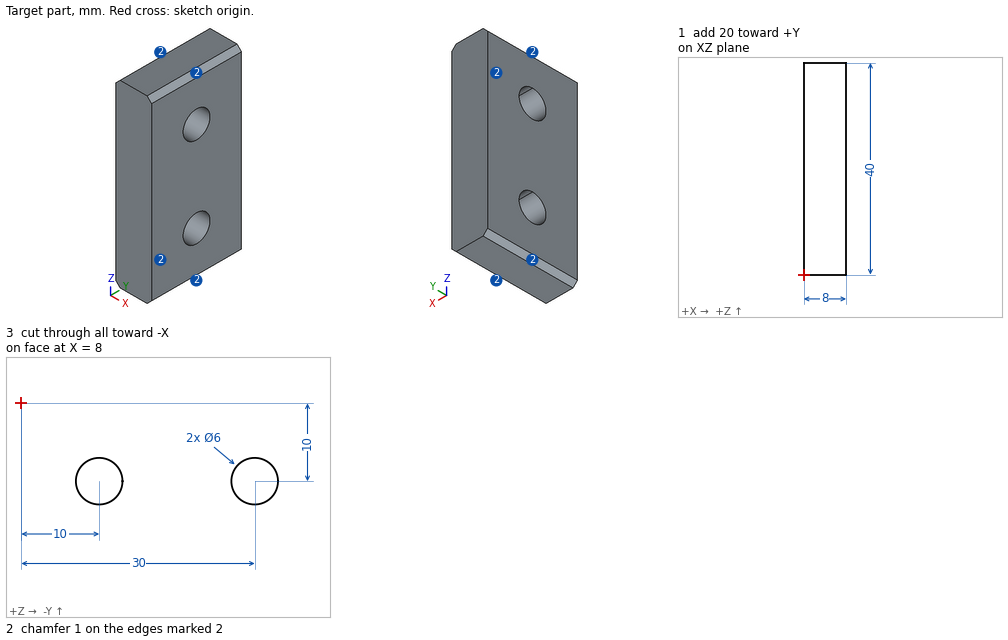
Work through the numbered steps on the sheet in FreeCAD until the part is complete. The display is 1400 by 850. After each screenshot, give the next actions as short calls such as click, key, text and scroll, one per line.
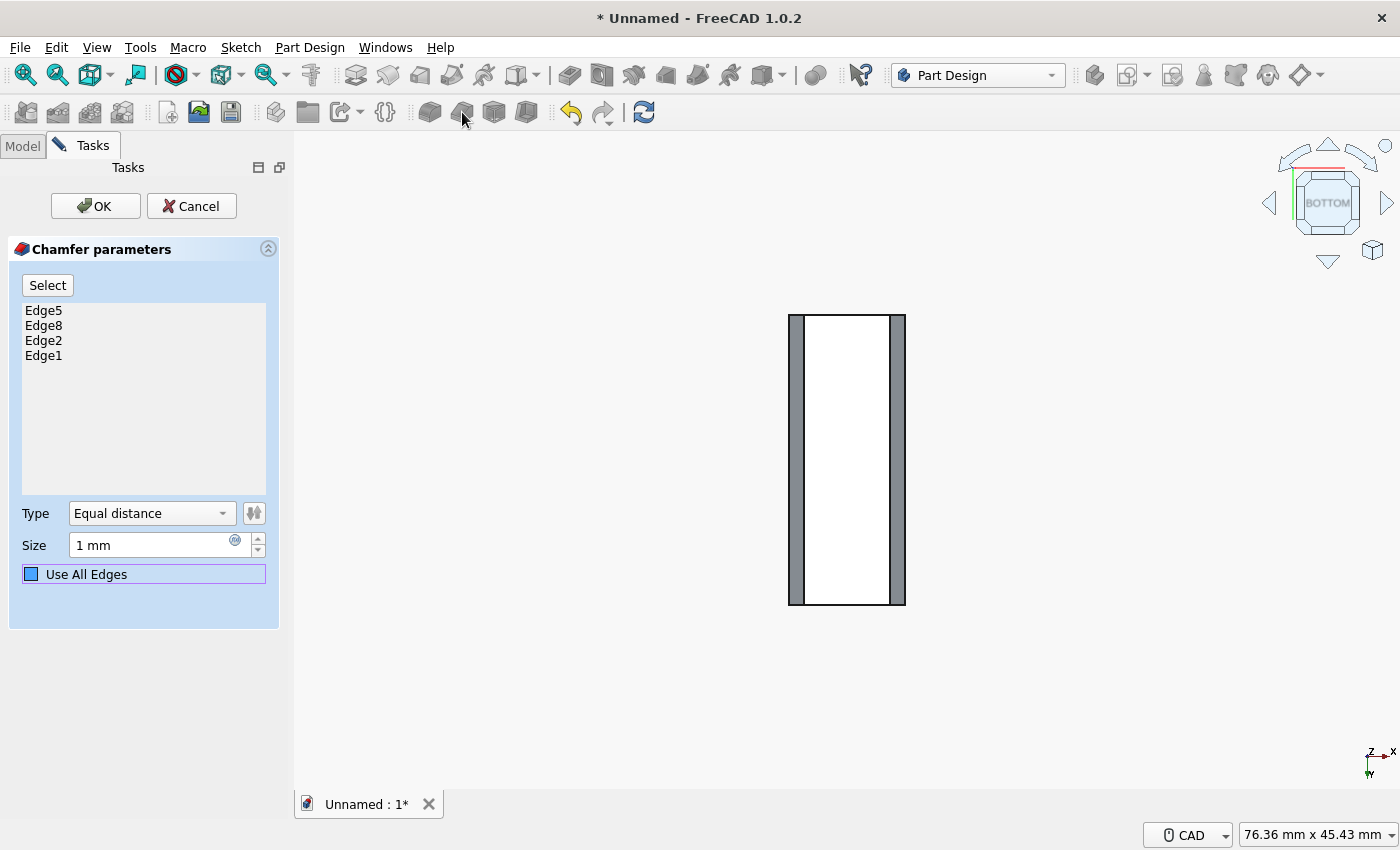
click(96, 206)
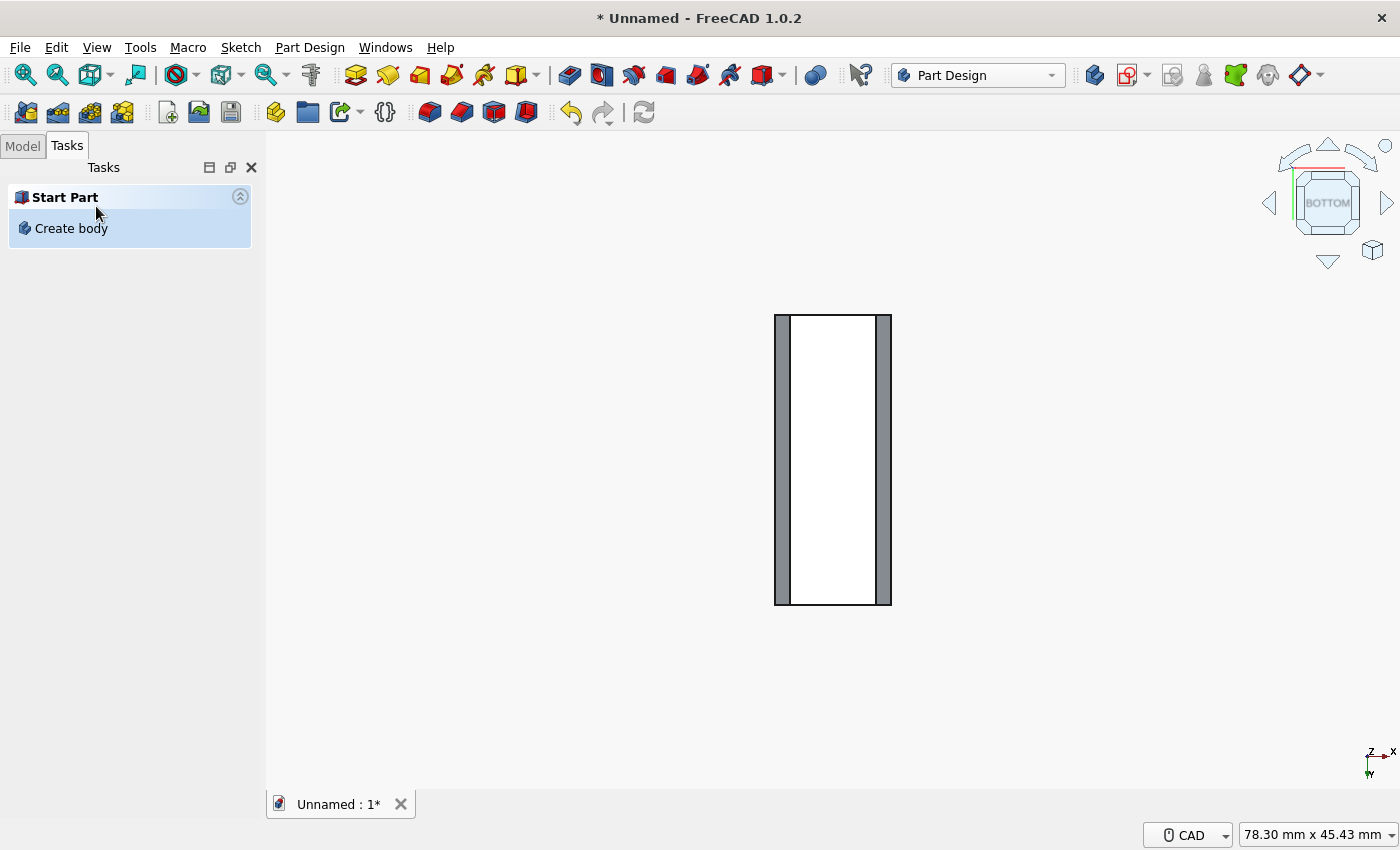
click(26, 76)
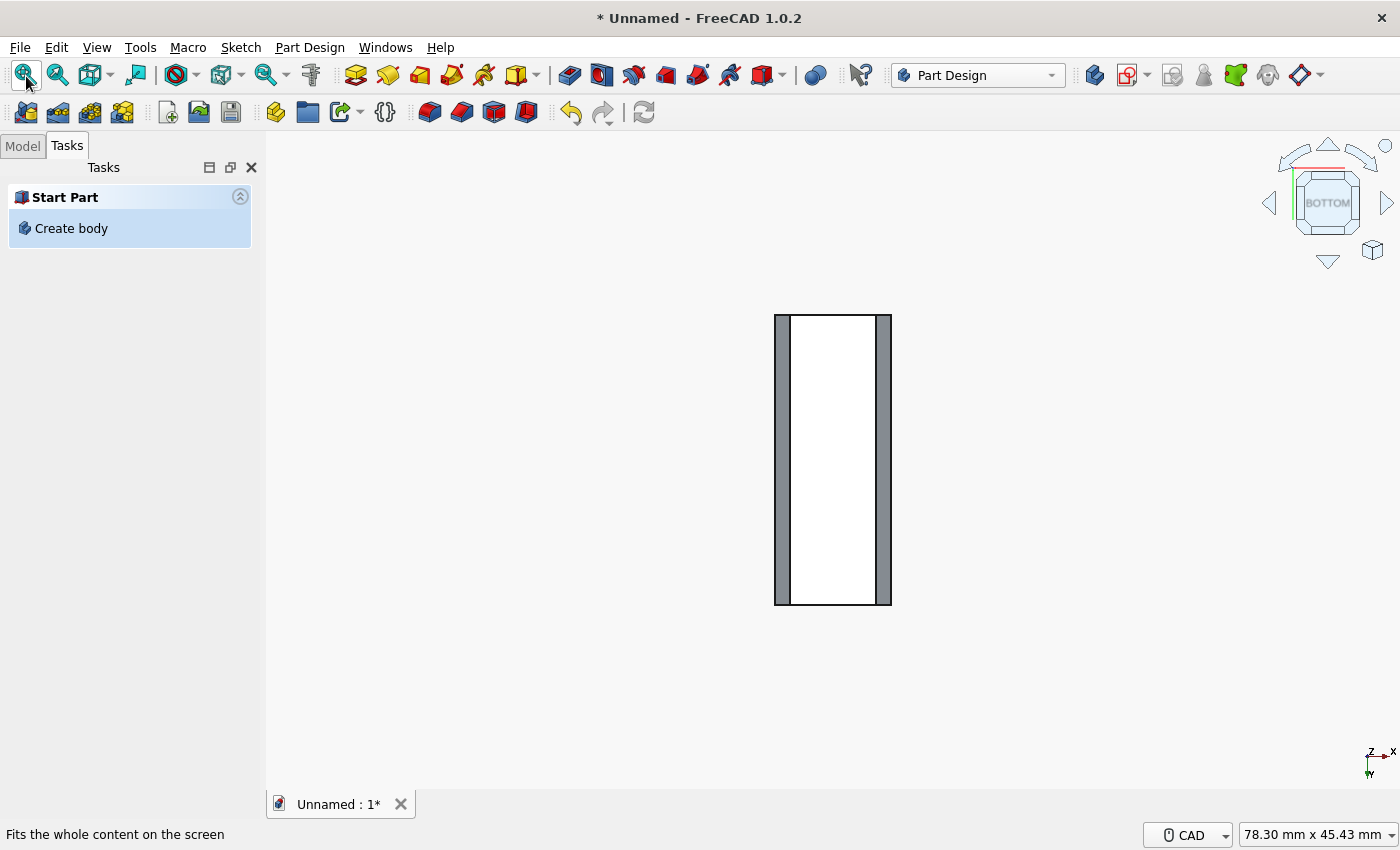
key(0)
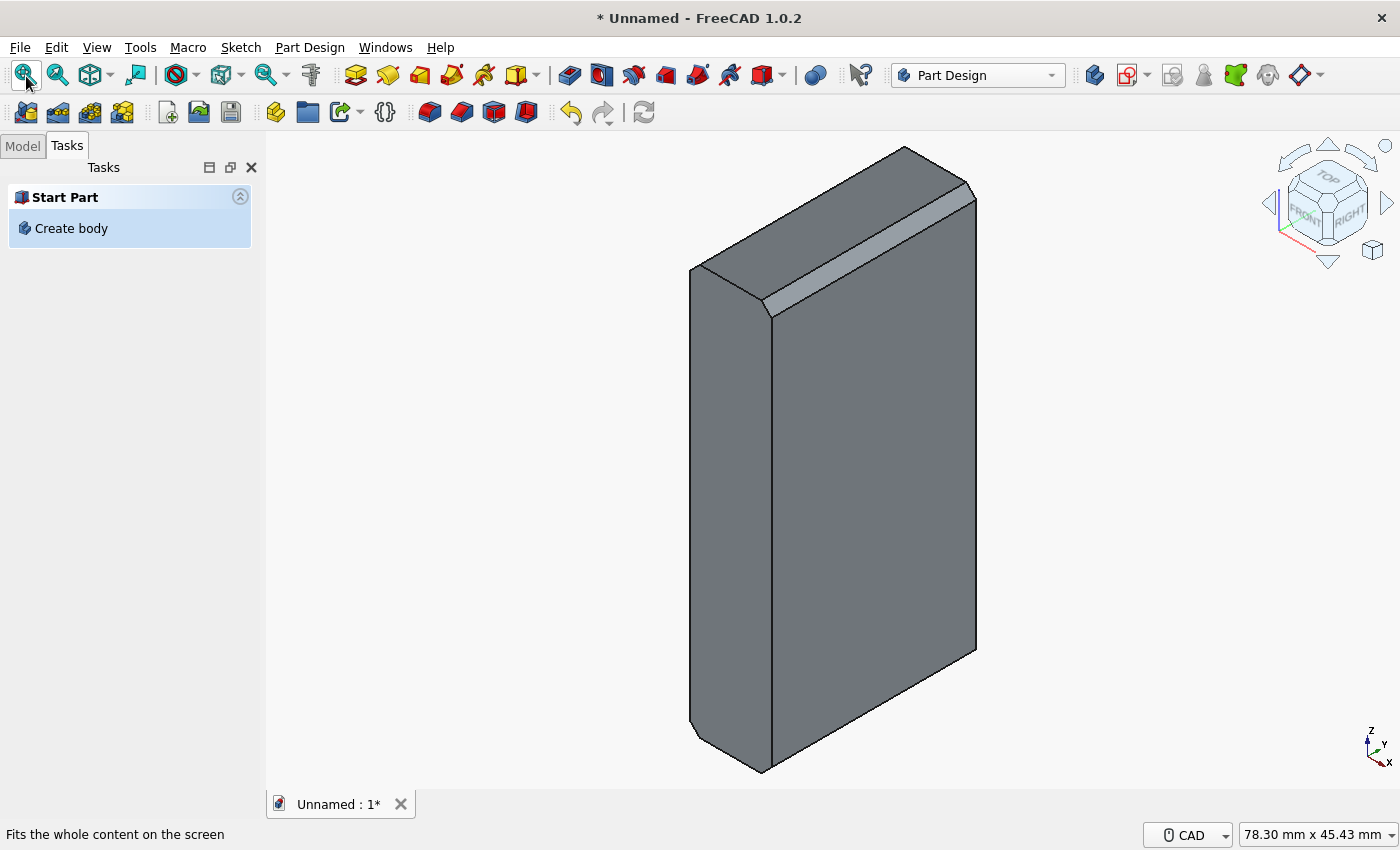
click(874, 418)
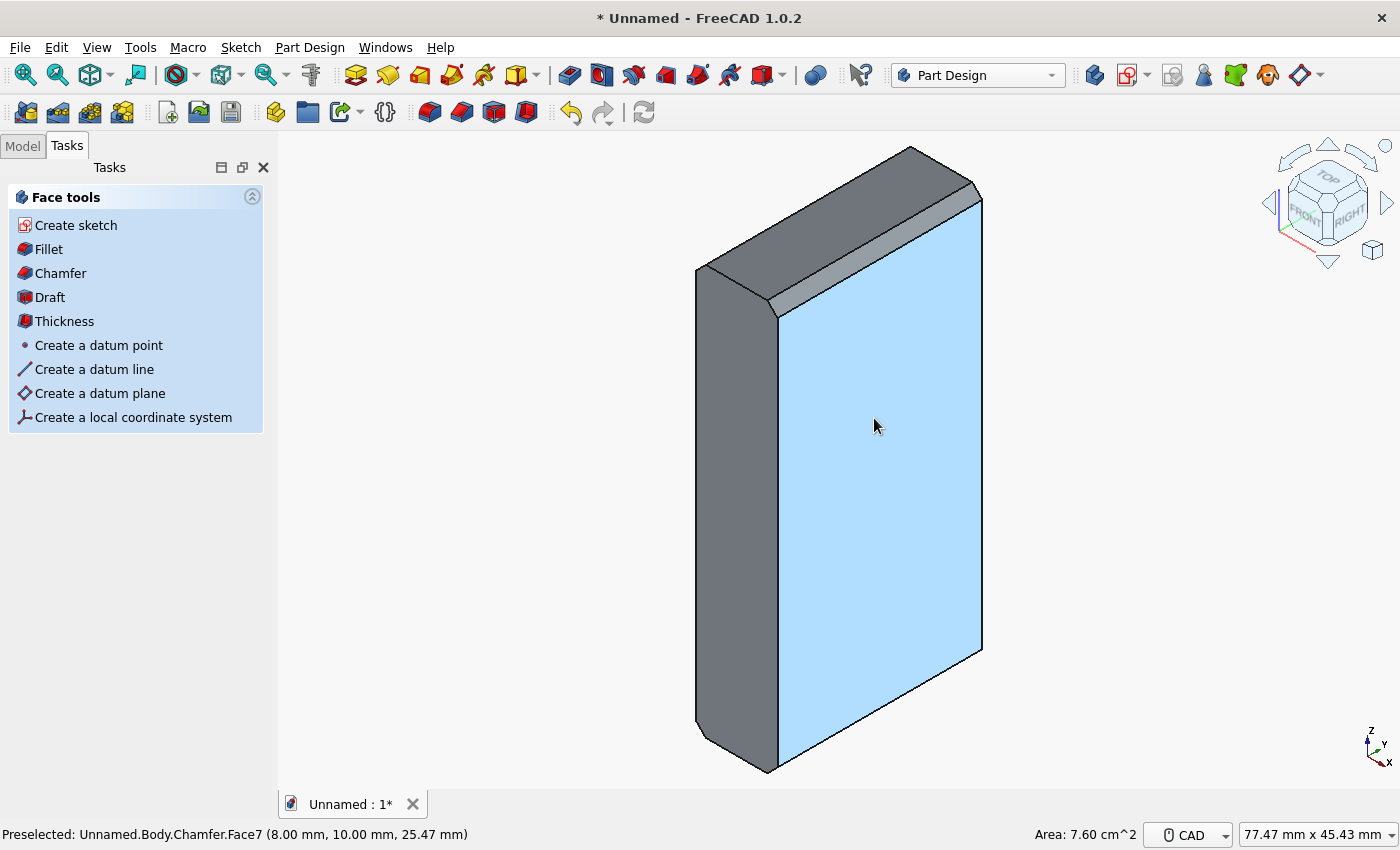
click(1128, 76)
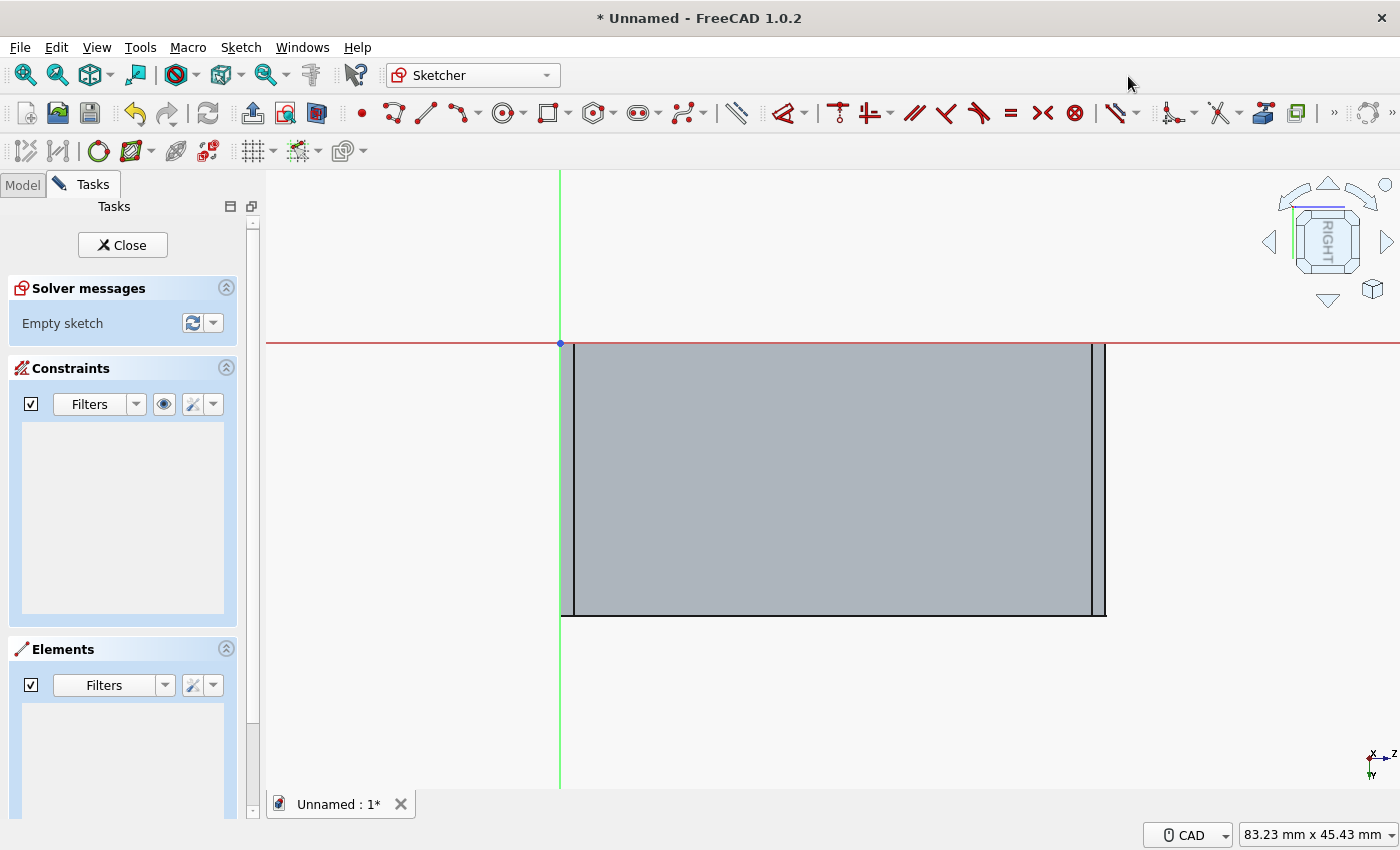
scroll(828, 335, up, 2)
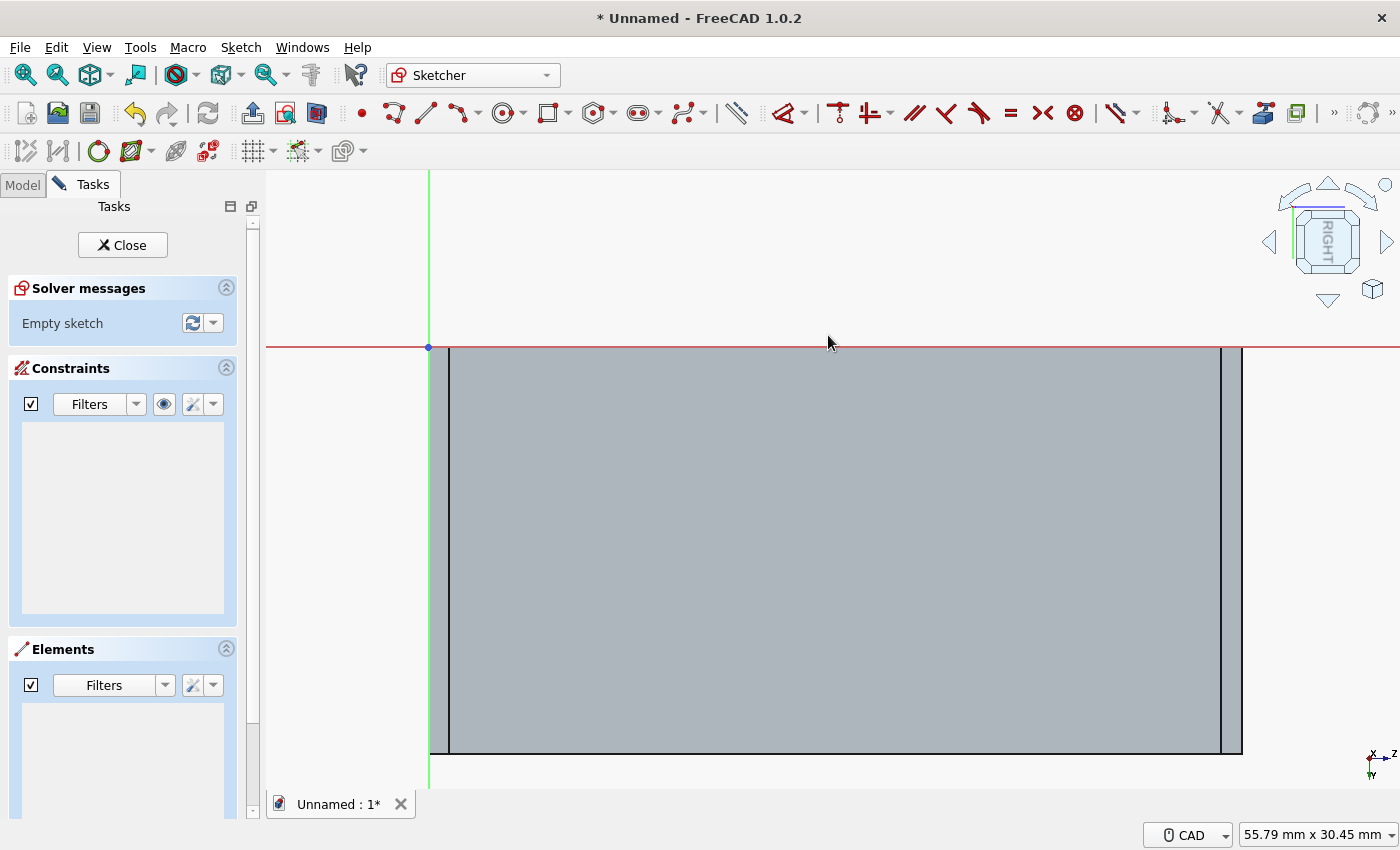
click(504, 114)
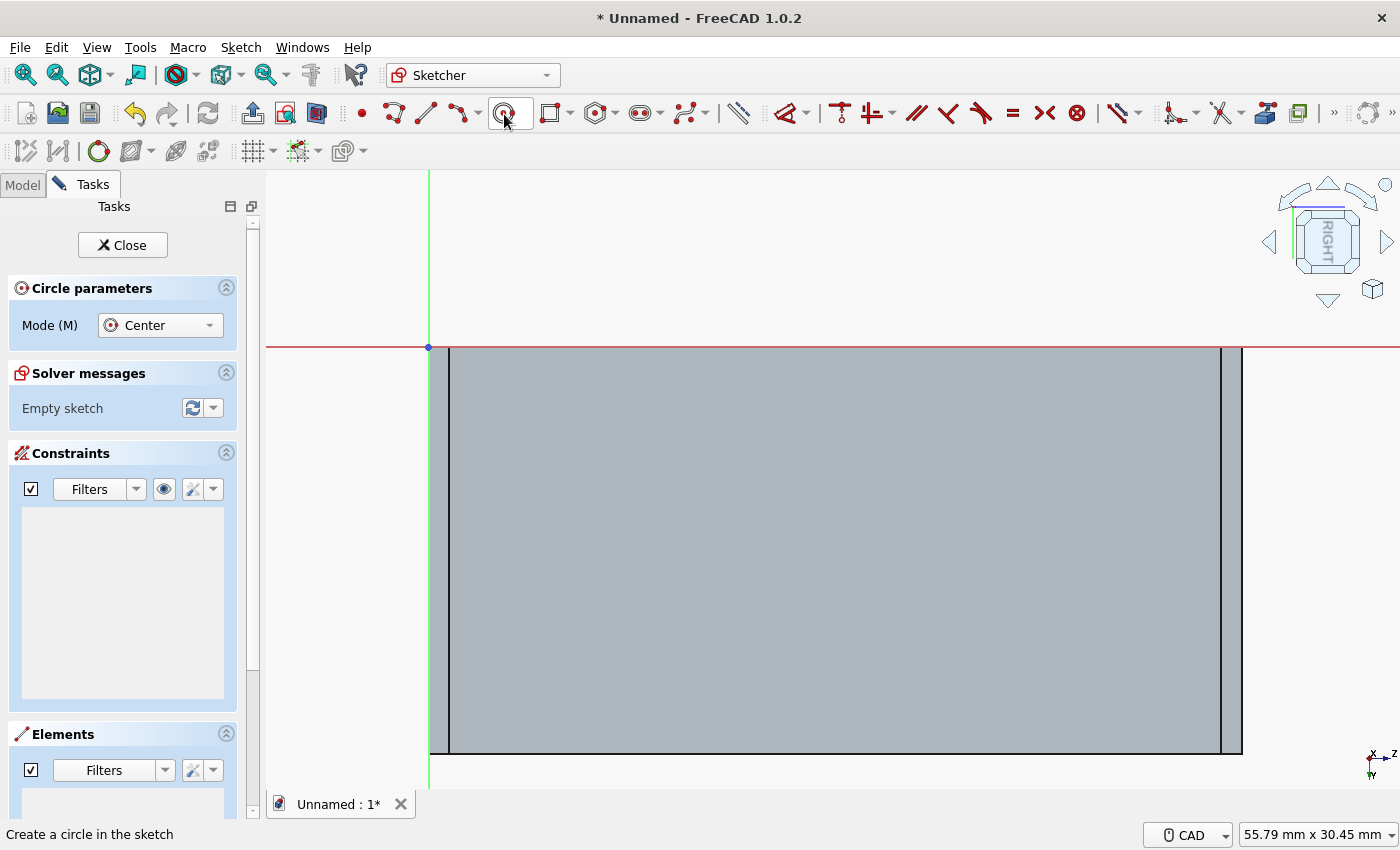
click(1038, 550)
move(1082, 507)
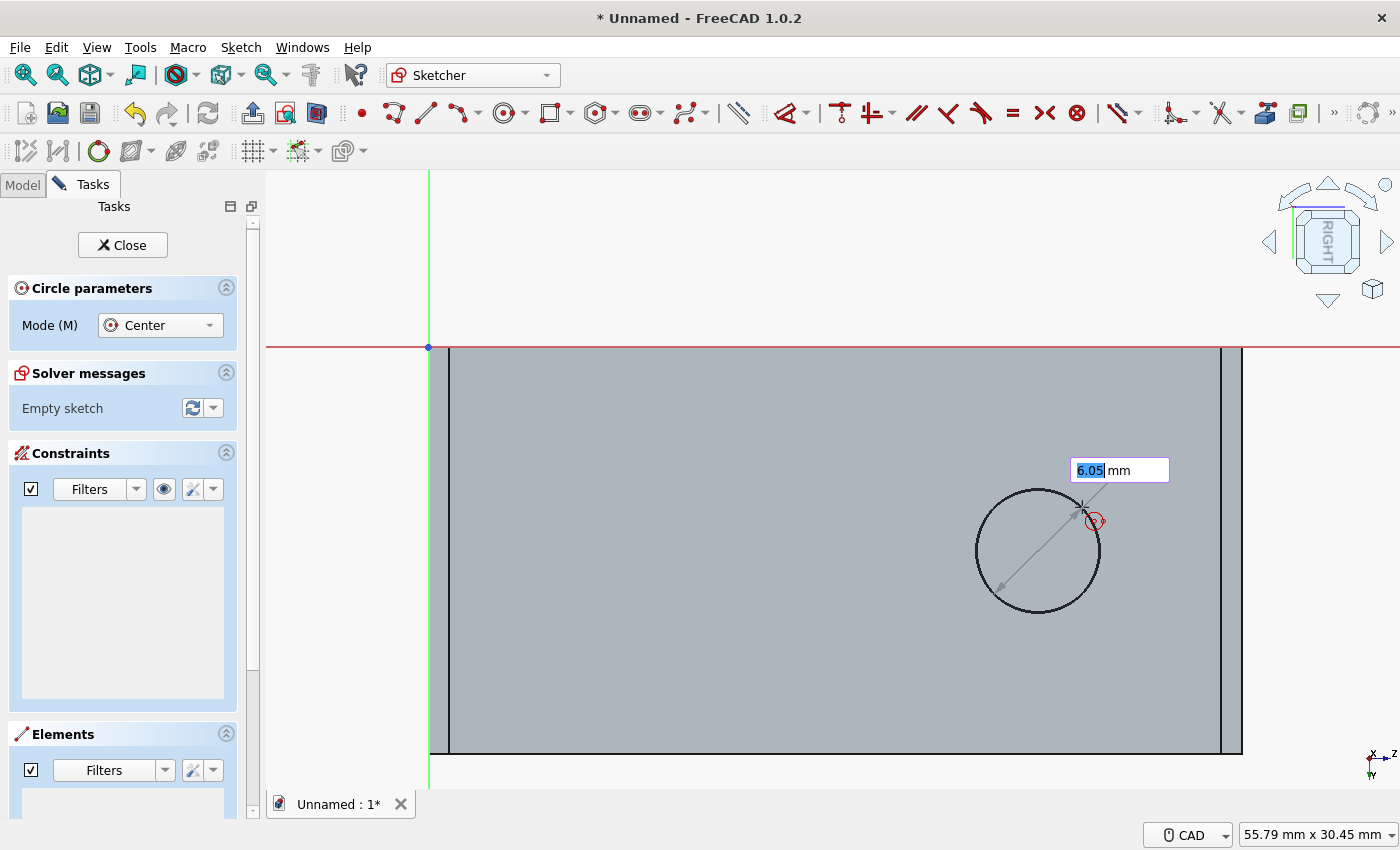
text(6)
key(Return)